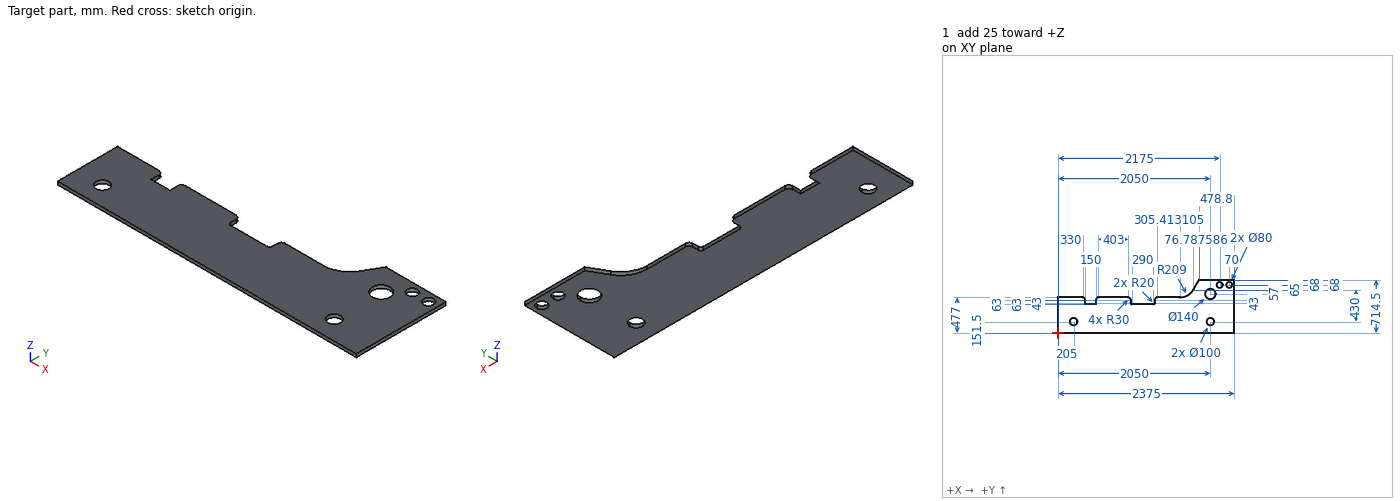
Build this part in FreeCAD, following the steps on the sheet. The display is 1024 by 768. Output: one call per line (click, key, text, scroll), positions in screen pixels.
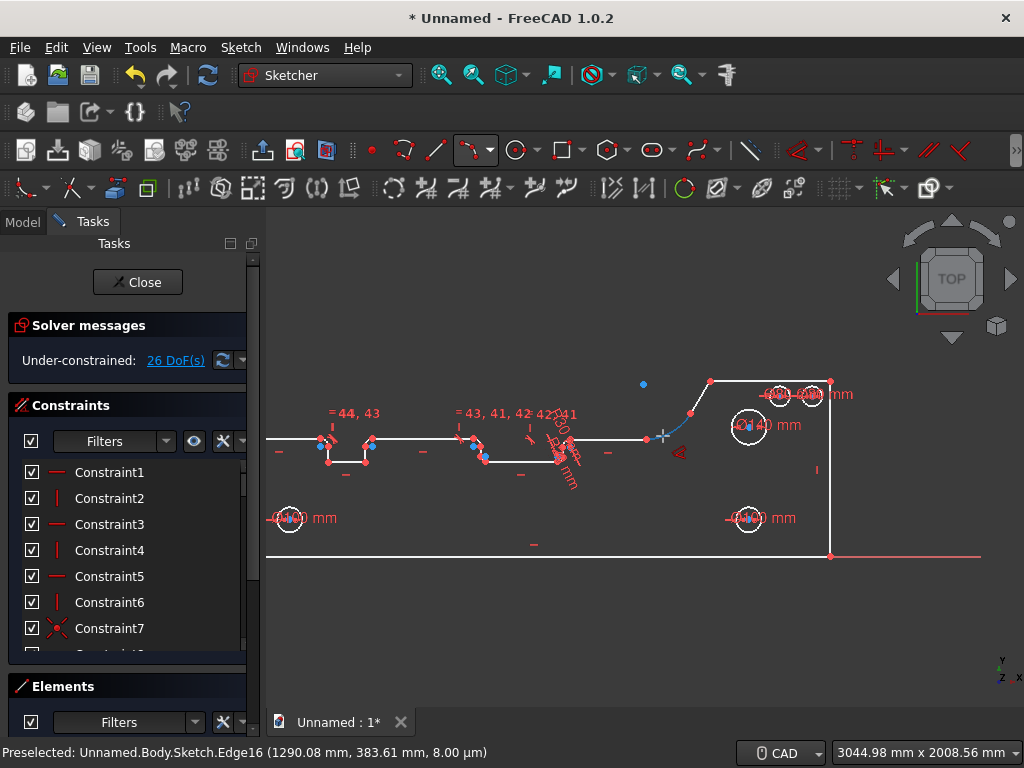
click(662, 436)
click(673, 466)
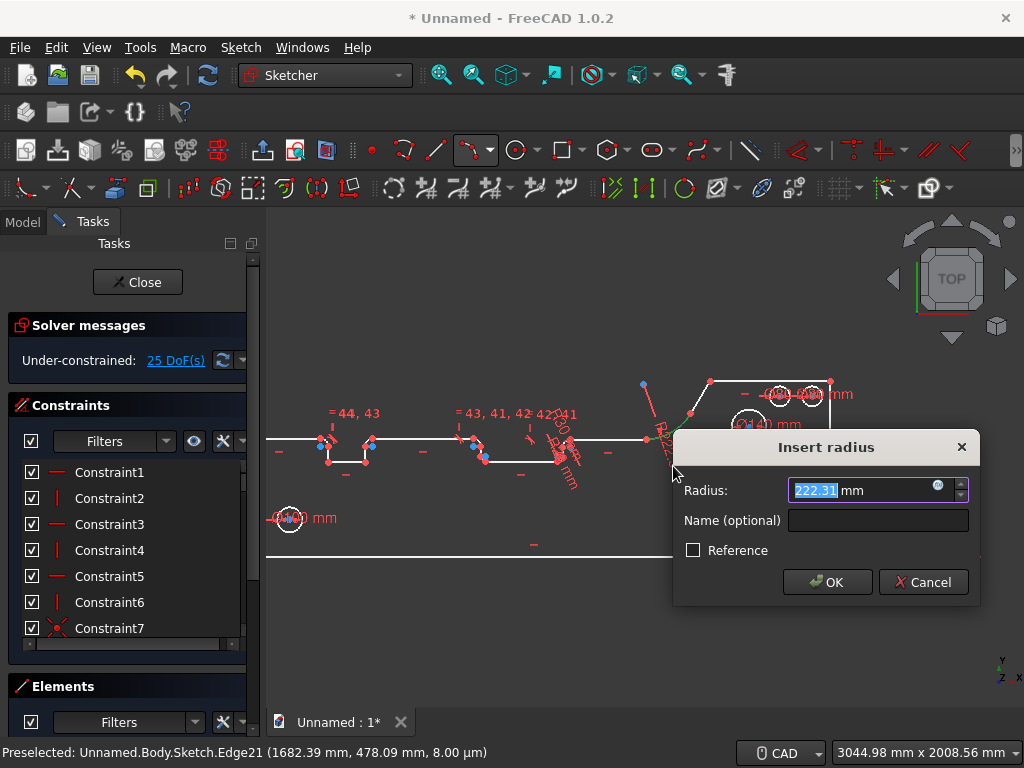
text(209)
key(Return)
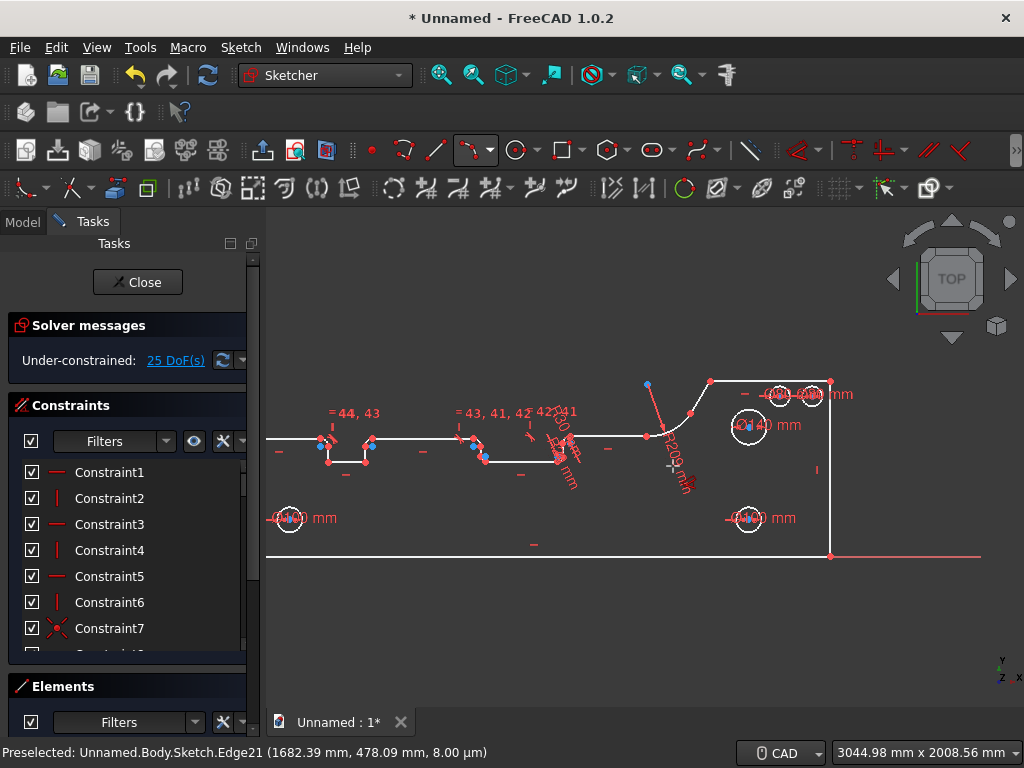
scroll(563, 450, up, 7)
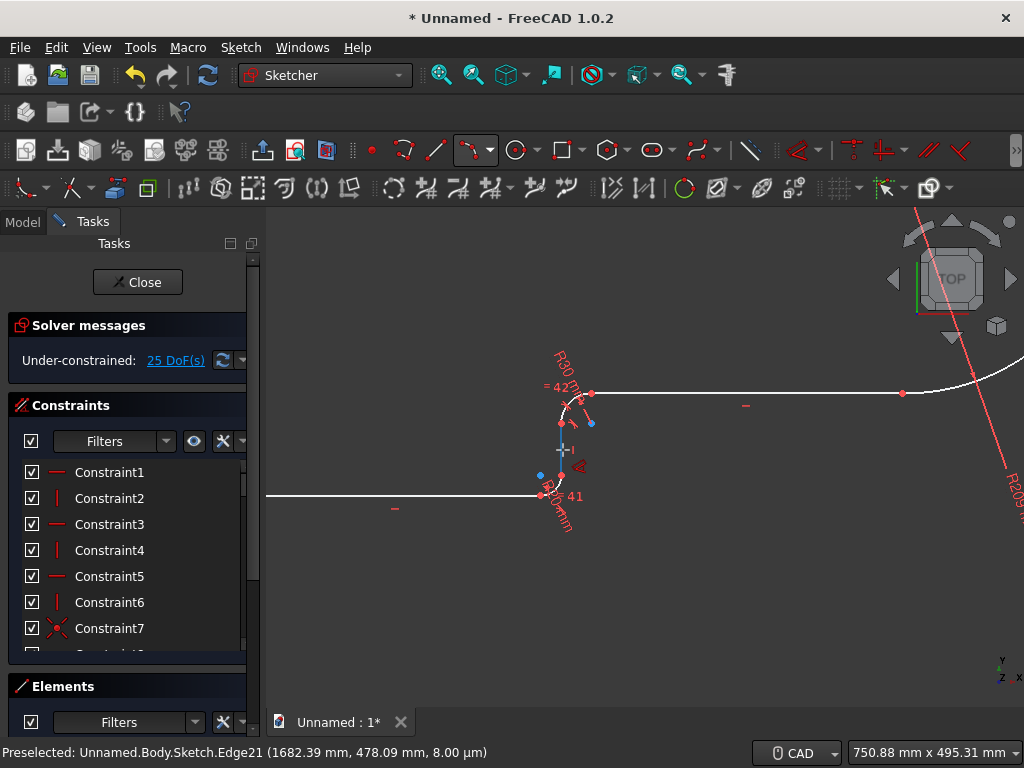
click(561, 450)
click(595, 450)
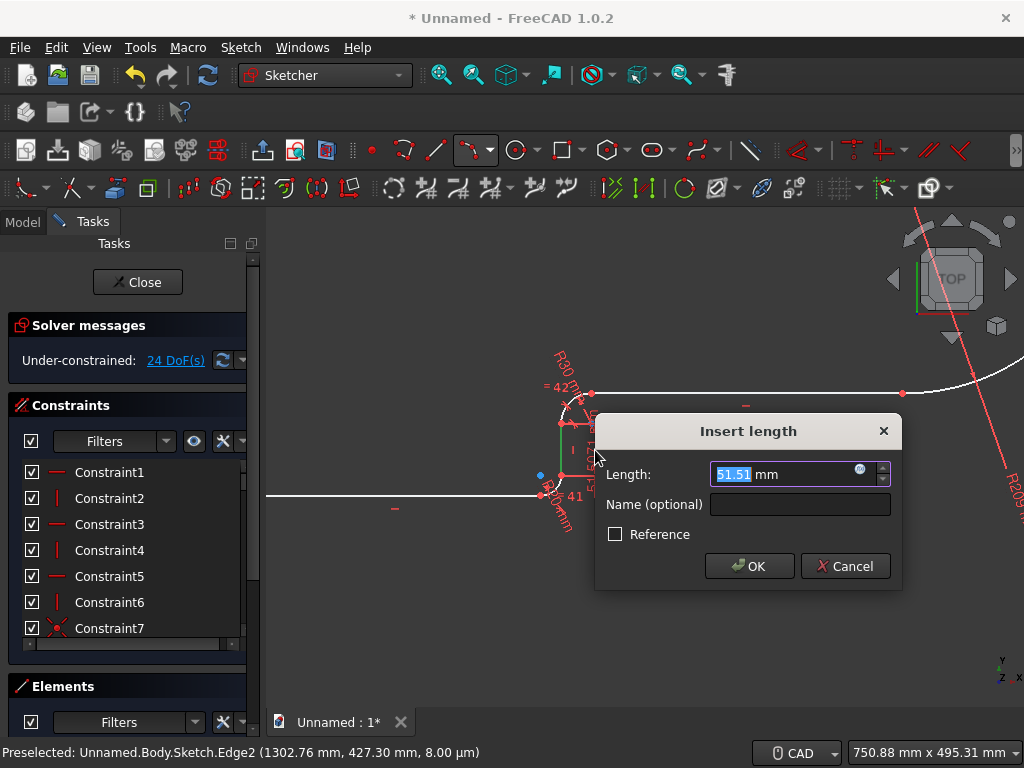
text(43)
key(Return)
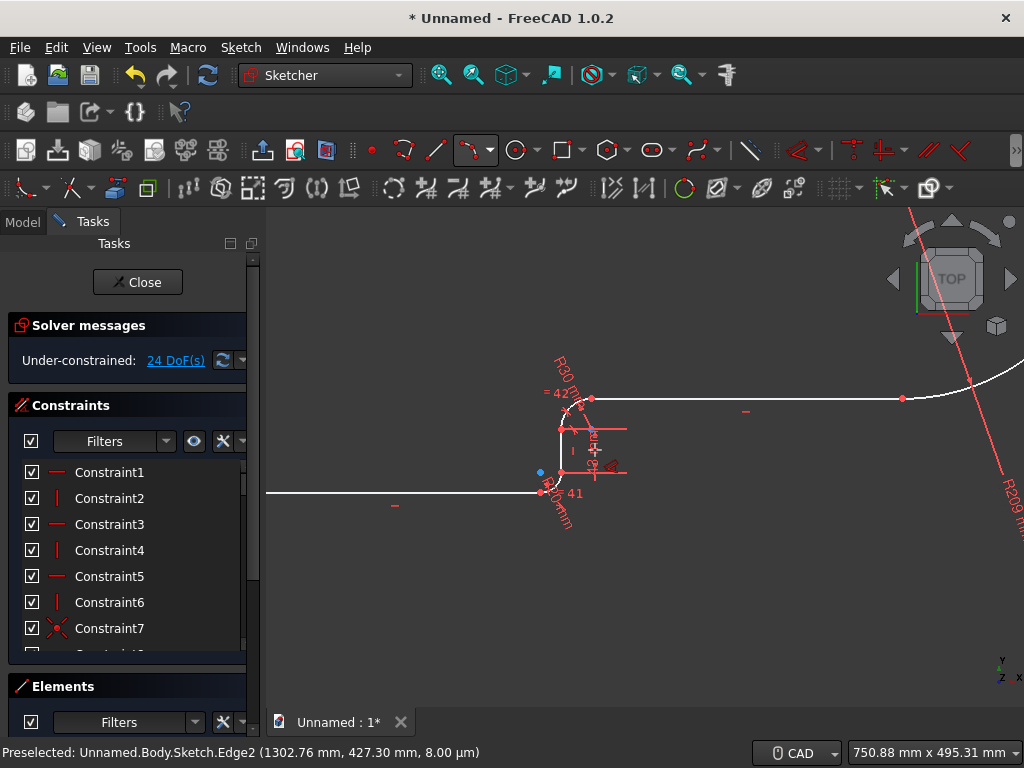
scroll(603, 444, down, 9)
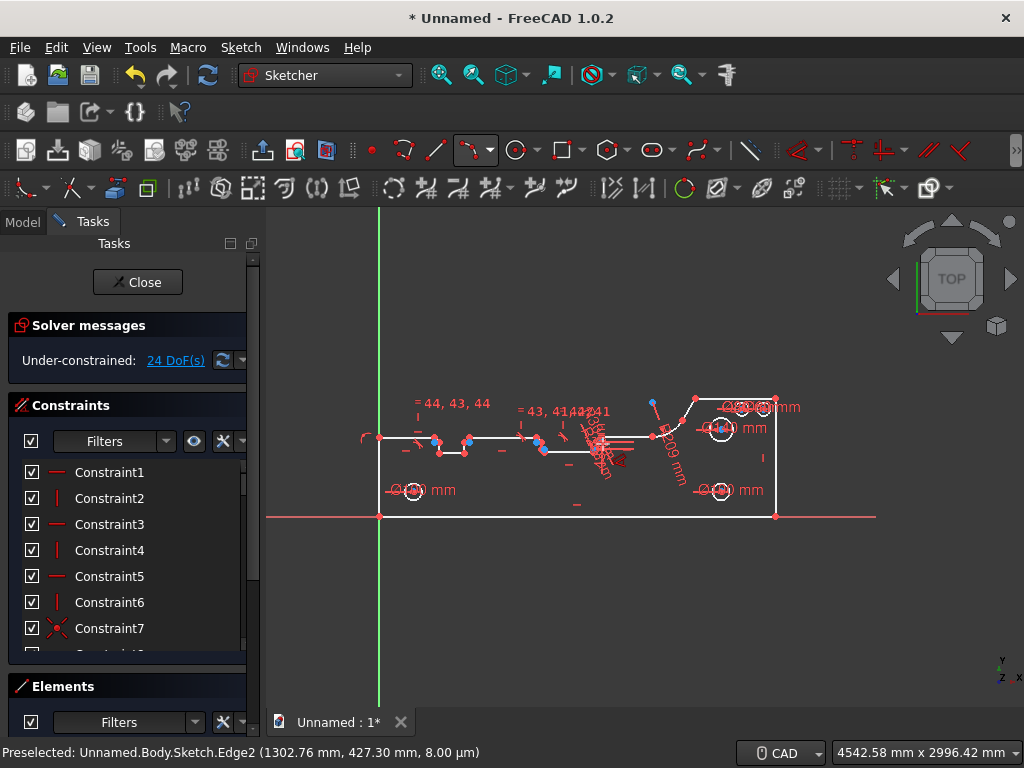
scroll(542, 447, up, 10)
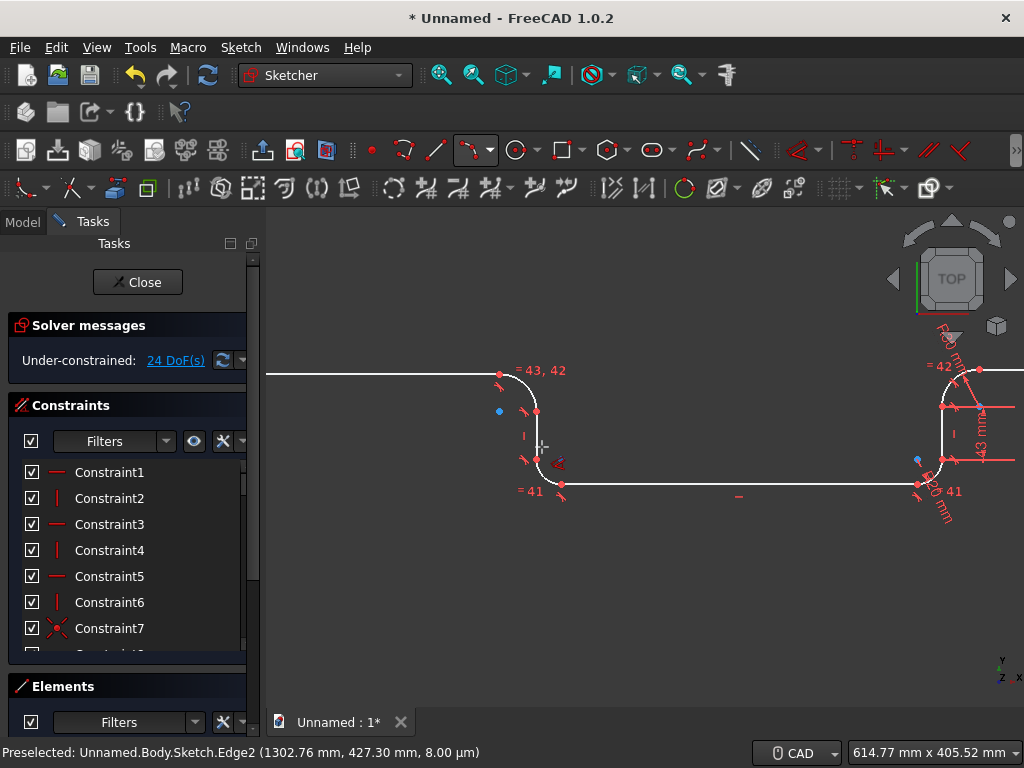
click(537, 445)
click(503, 435)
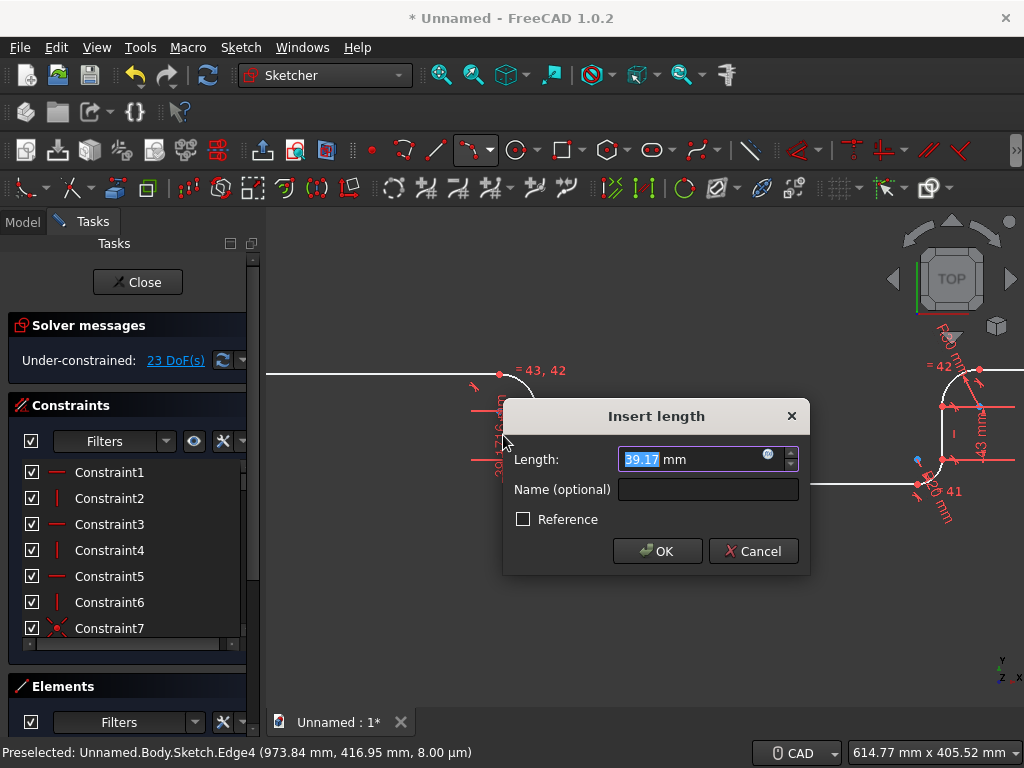
text(43)
key(Return)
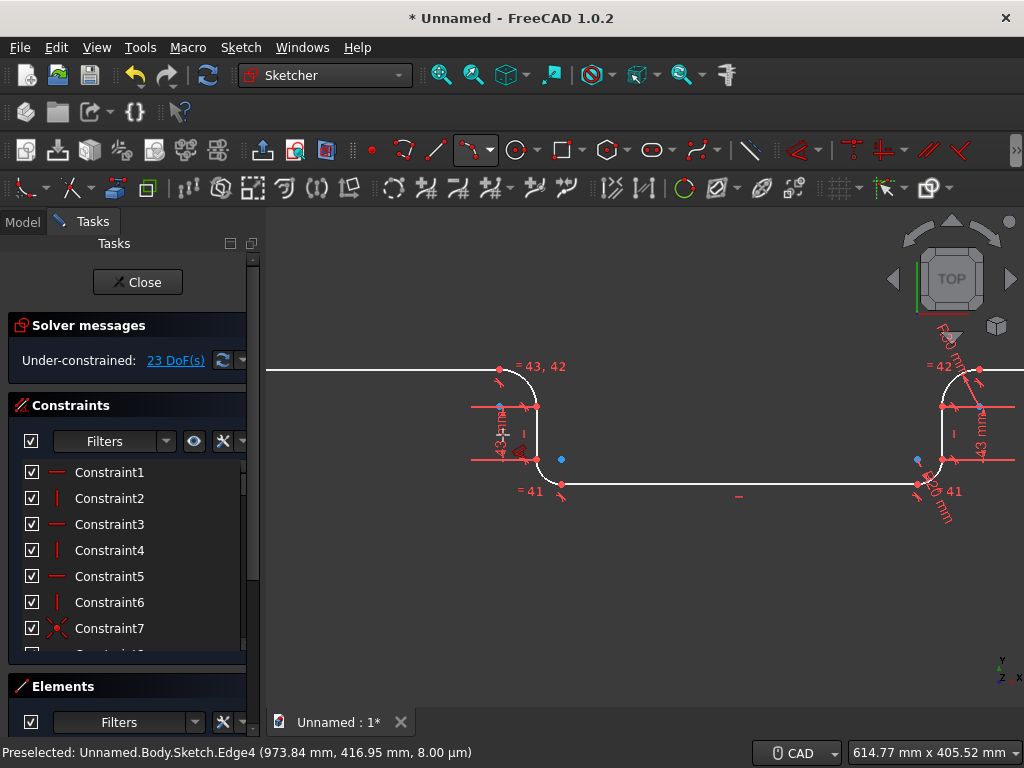
scroll(542, 447, down, 10)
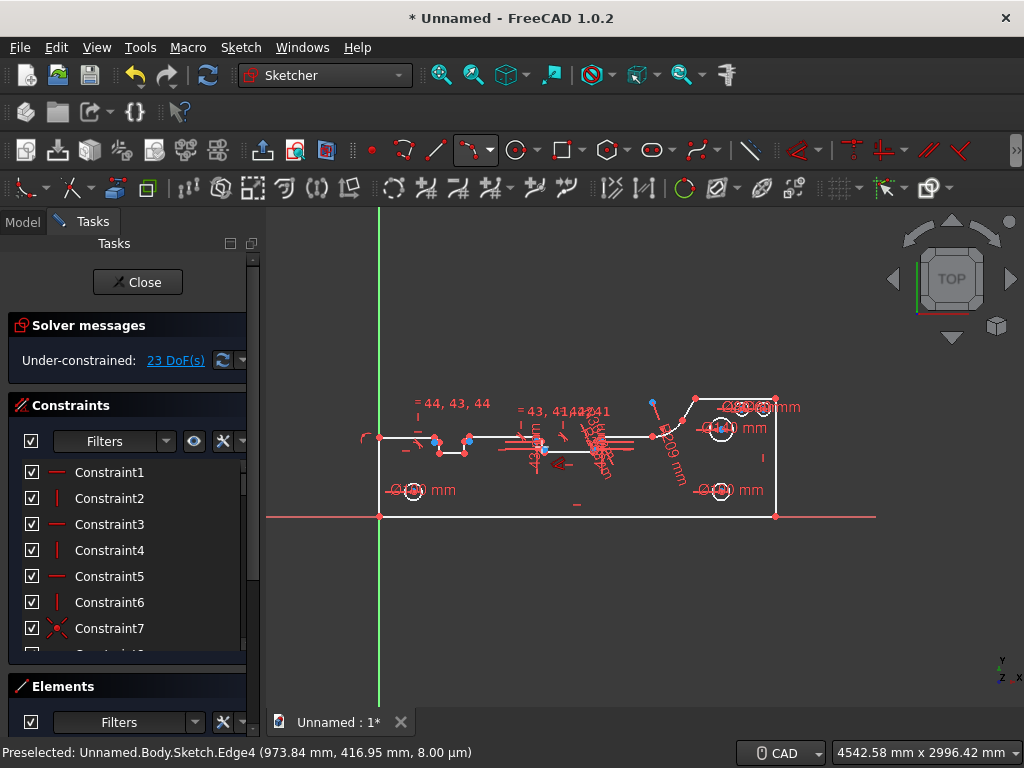
scroll(464, 445, up, 7)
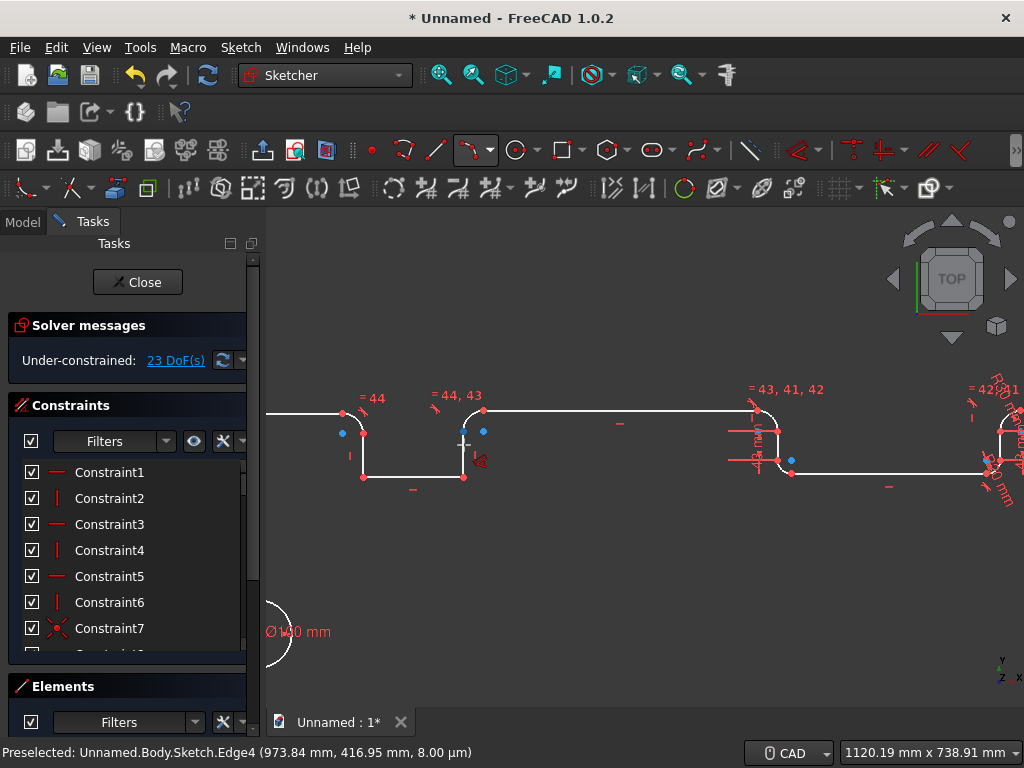
click(463, 445)
click(429, 454)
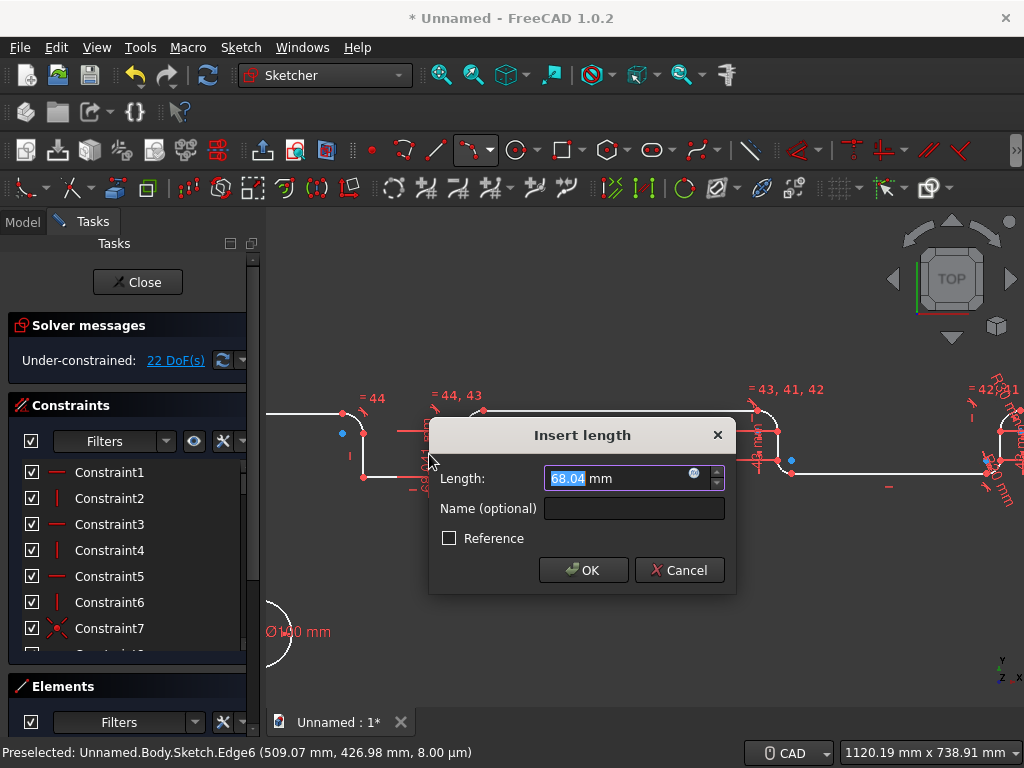
text(63)
key(Return)